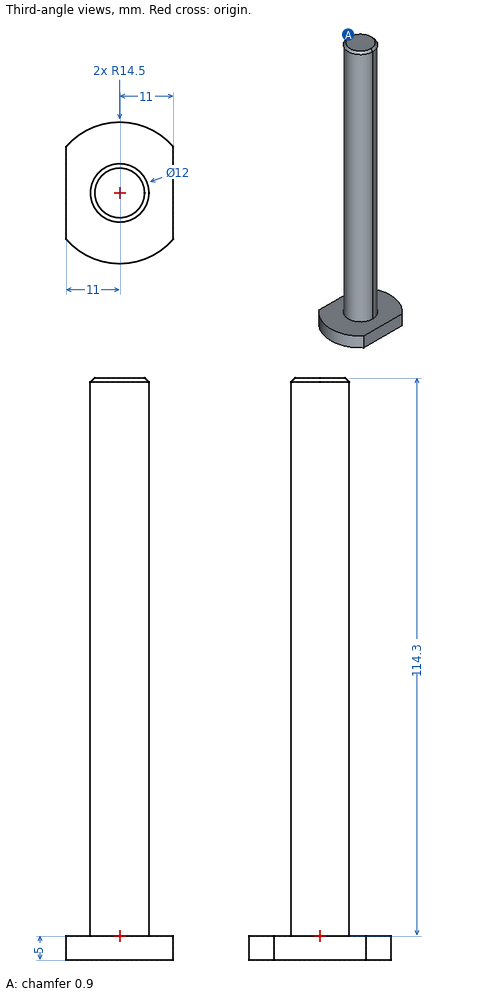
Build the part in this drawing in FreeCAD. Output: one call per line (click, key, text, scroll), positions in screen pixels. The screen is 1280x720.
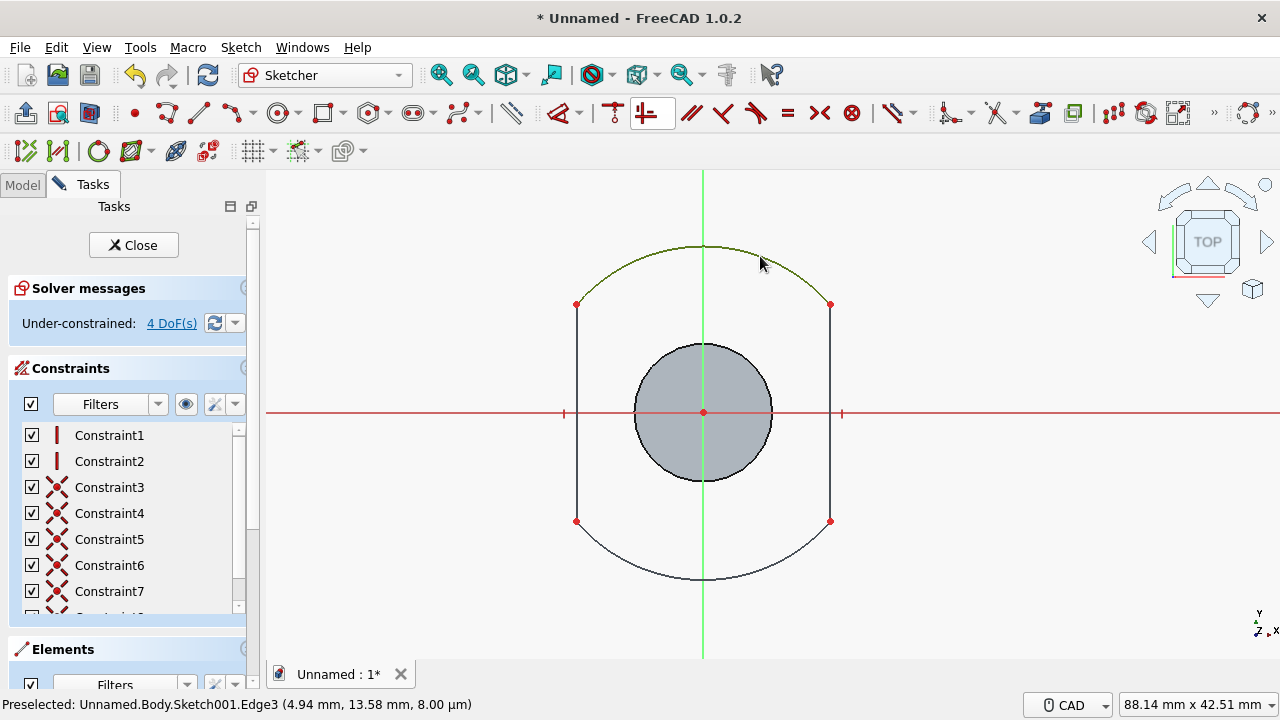
click(647, 570)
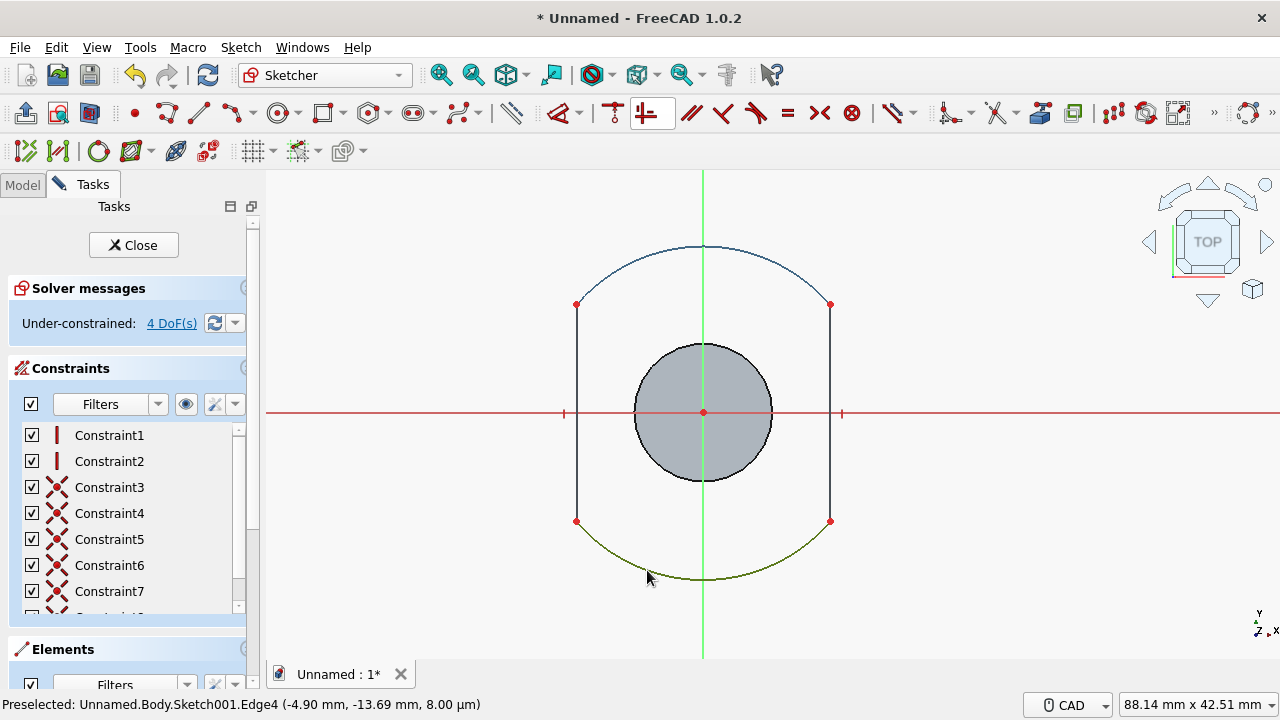
click(788, 114)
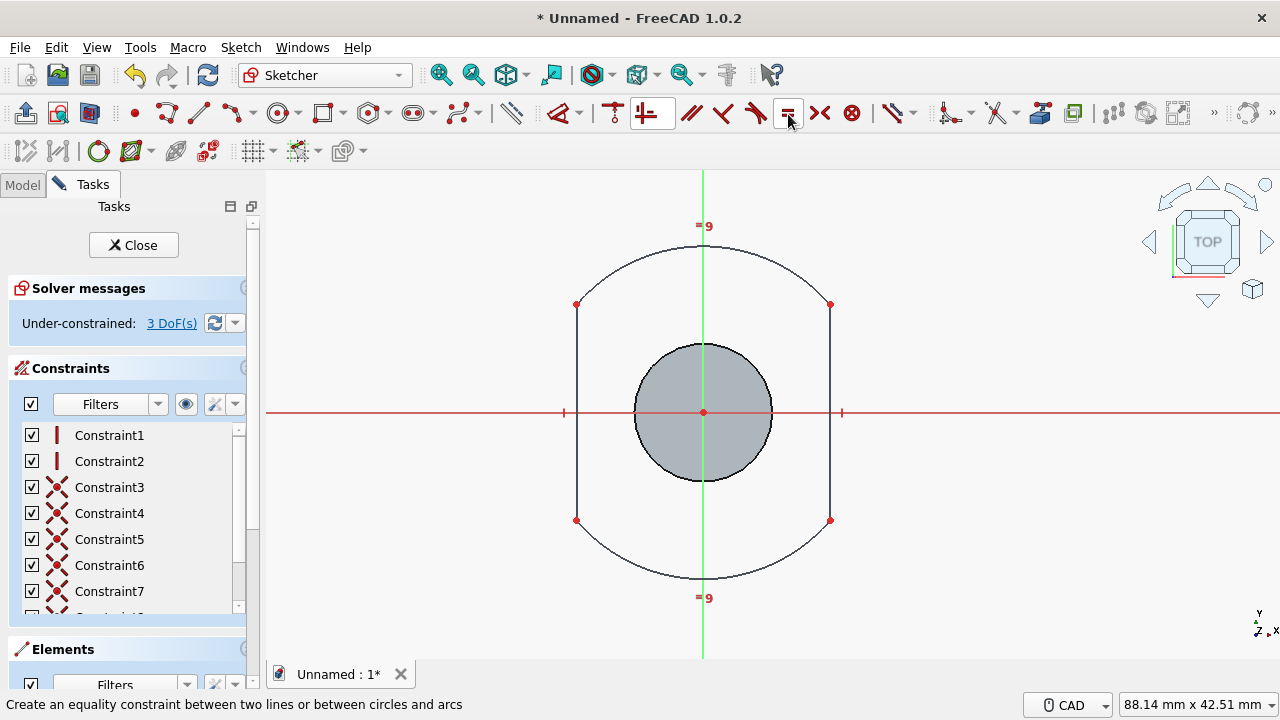
click(760, 256)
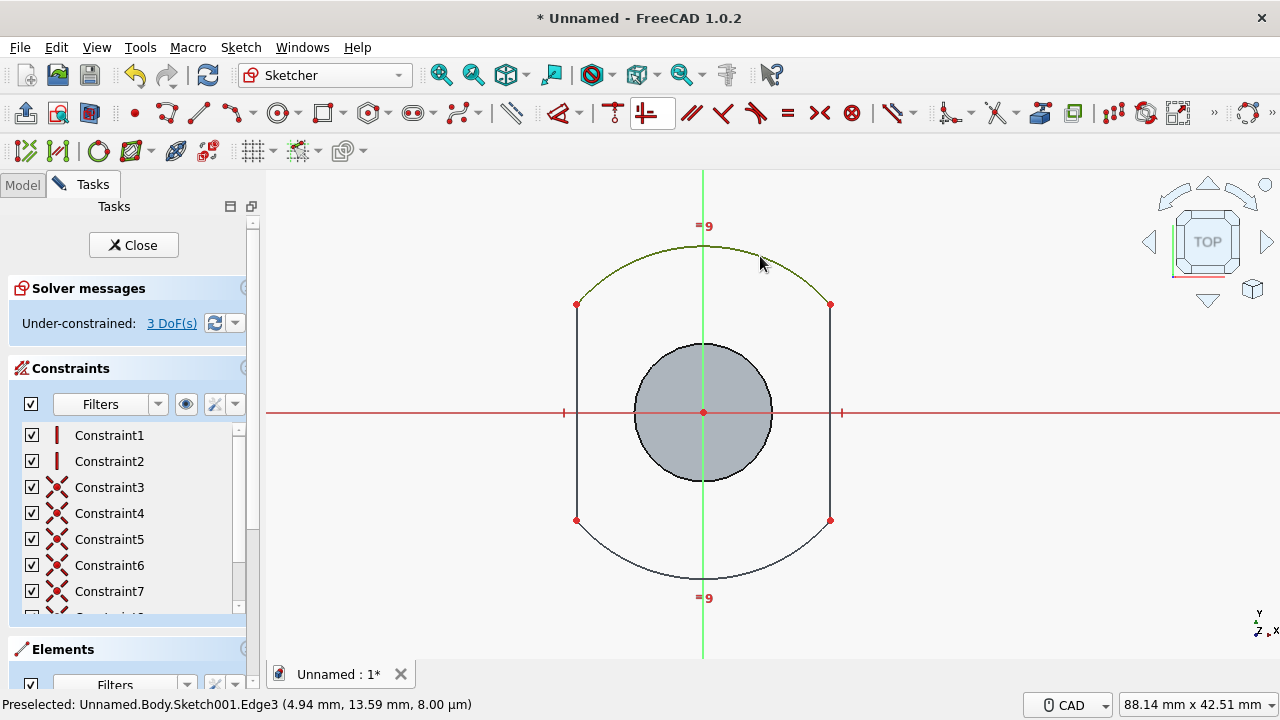
click(582, 114)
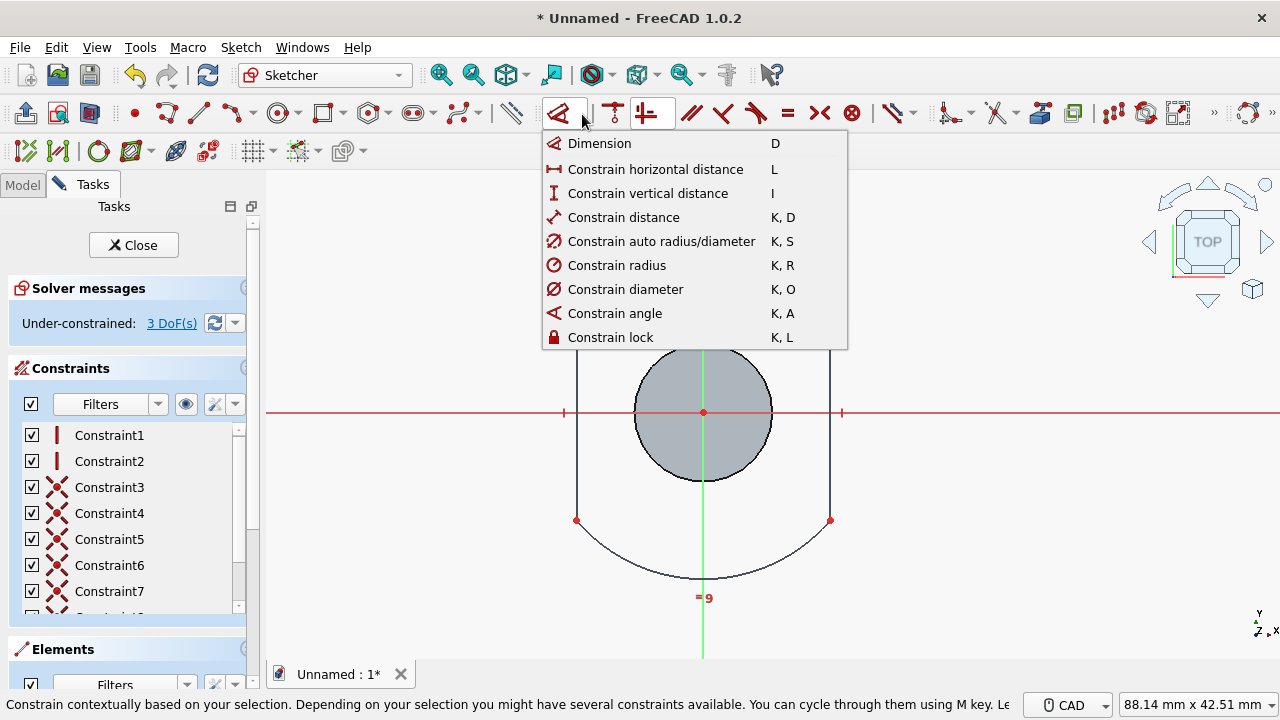
click(695, 265)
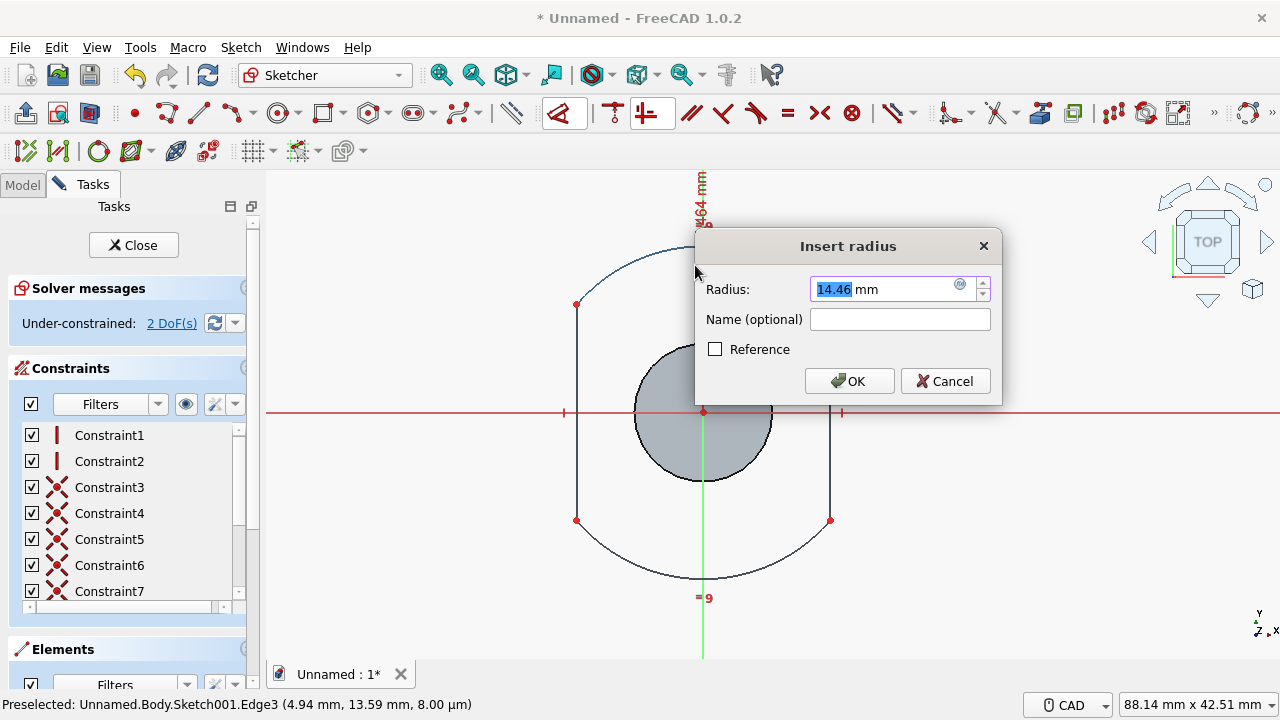
text(14.5)
key(Return)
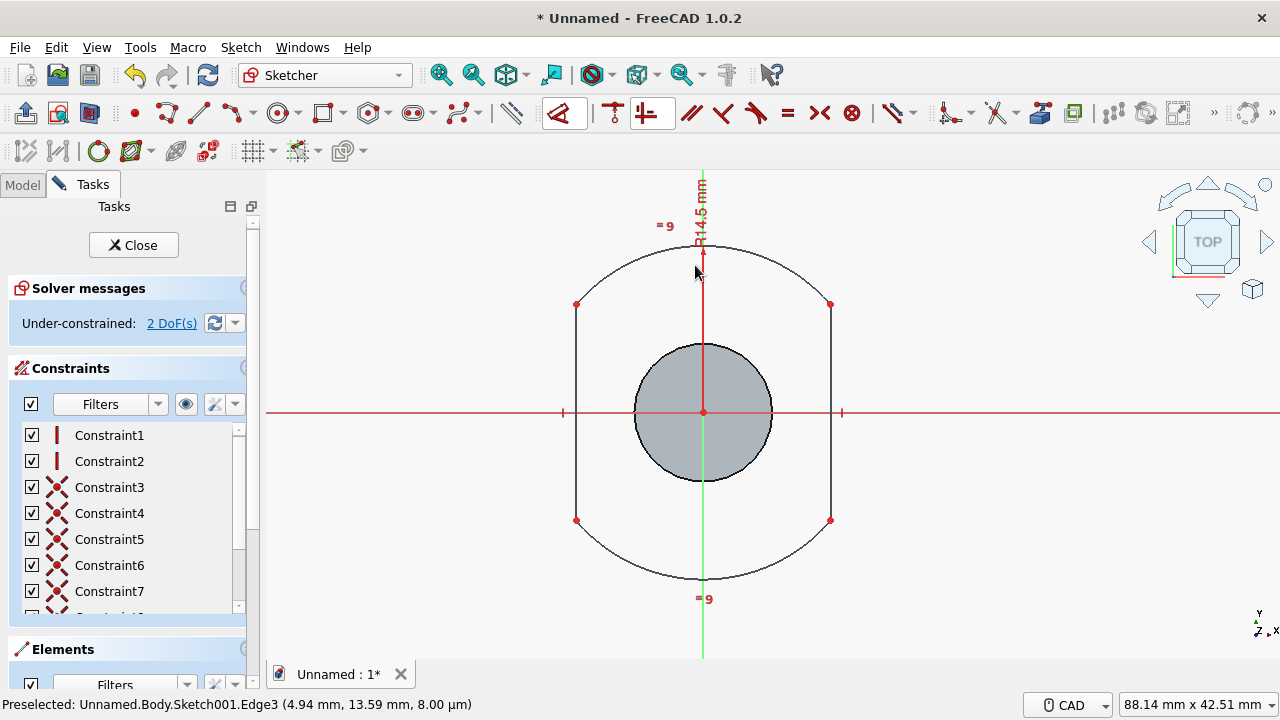
click(576, 521)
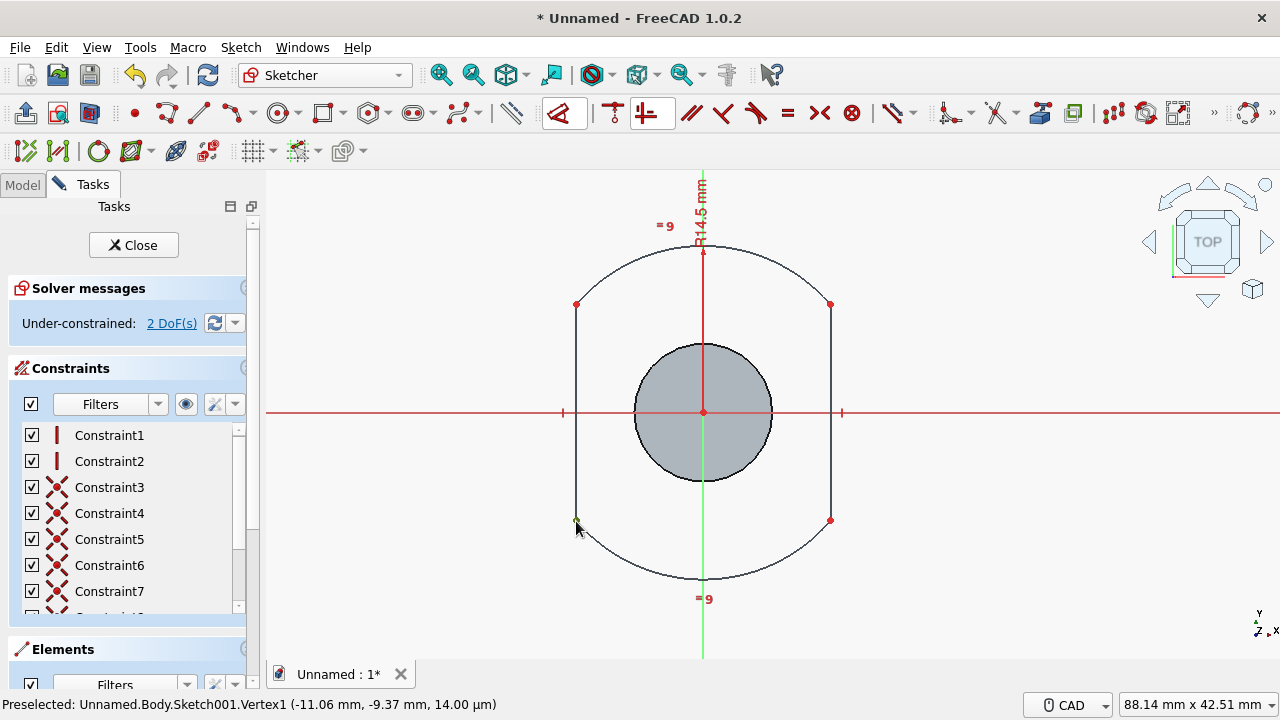
click(582, 114)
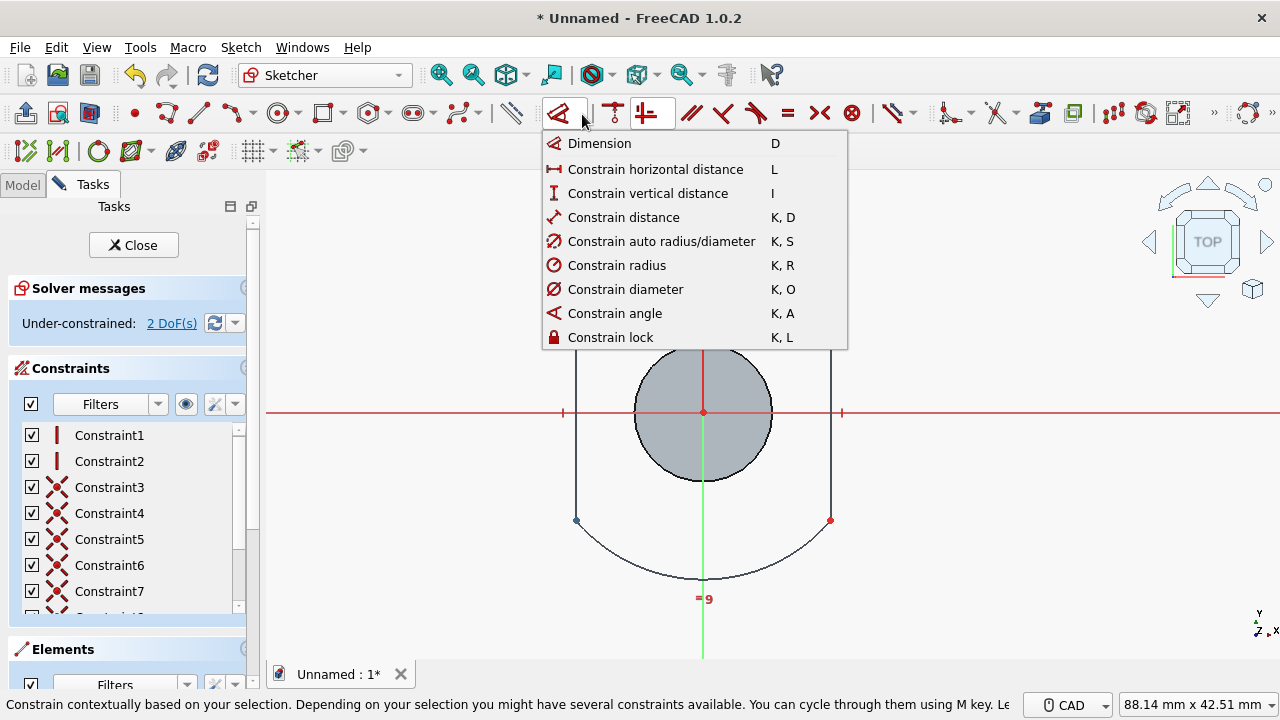
click(695, 169)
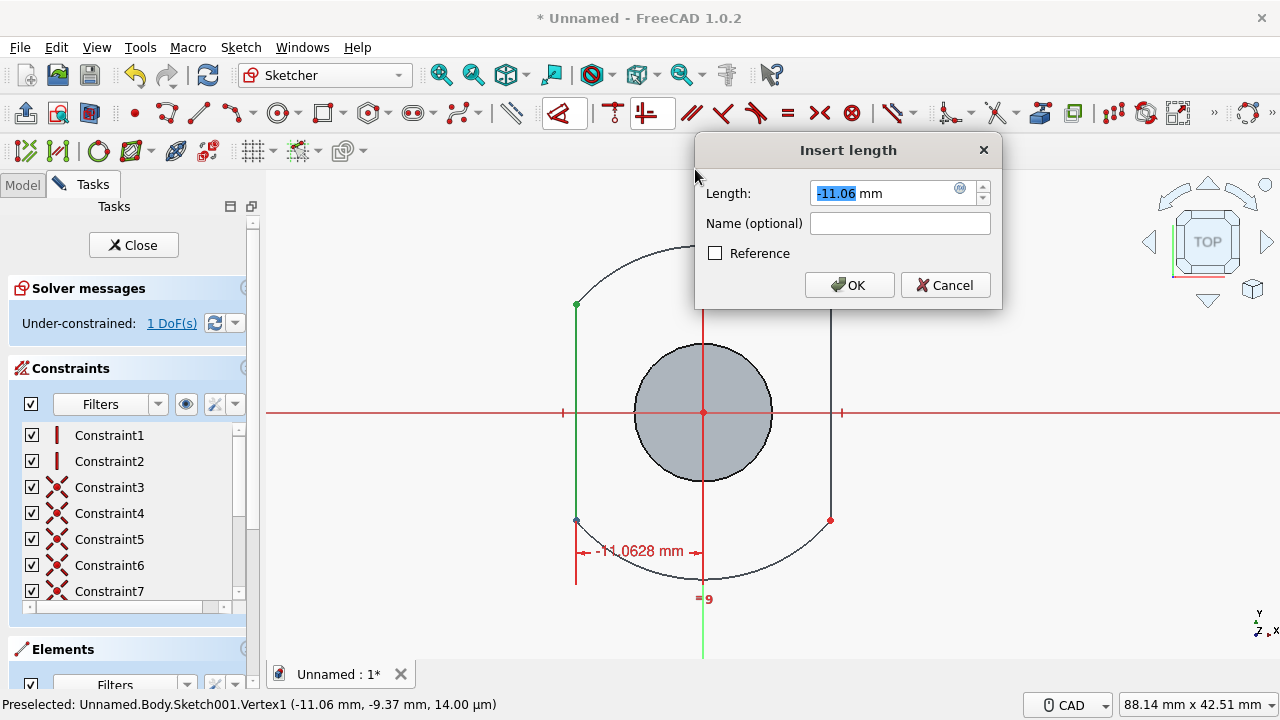
text(-11)
key(Return)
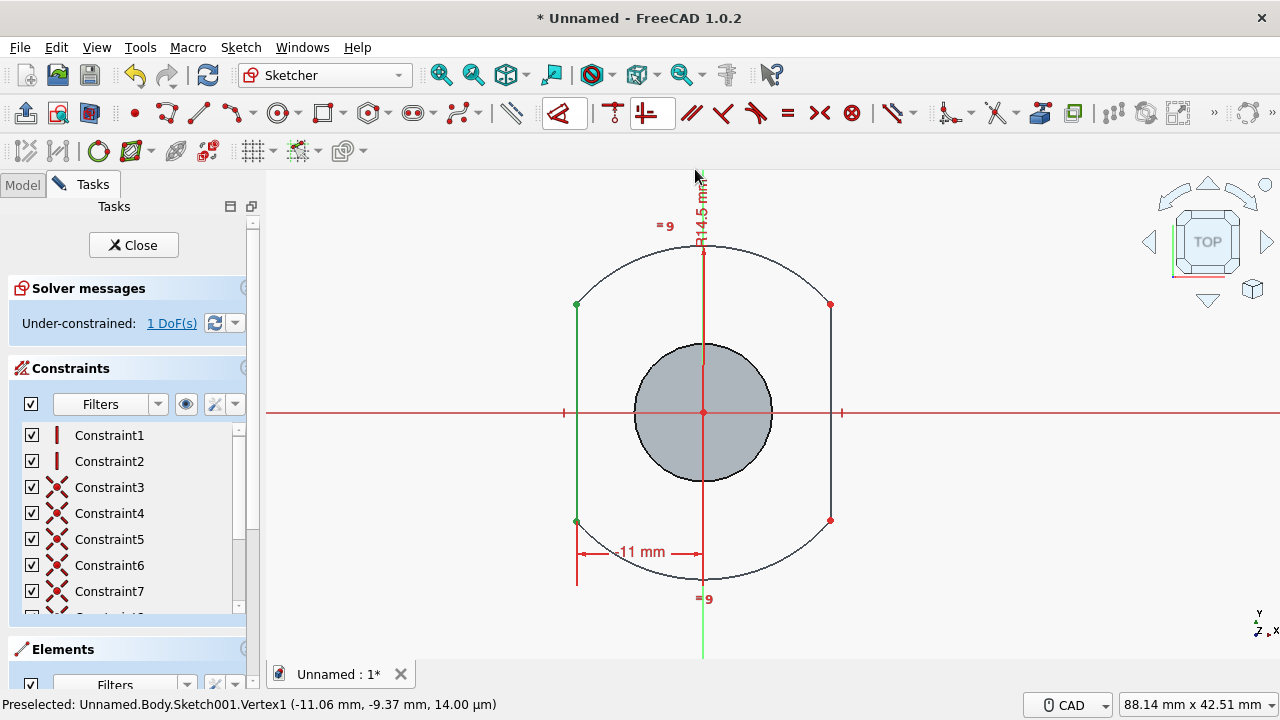
click(831, 305)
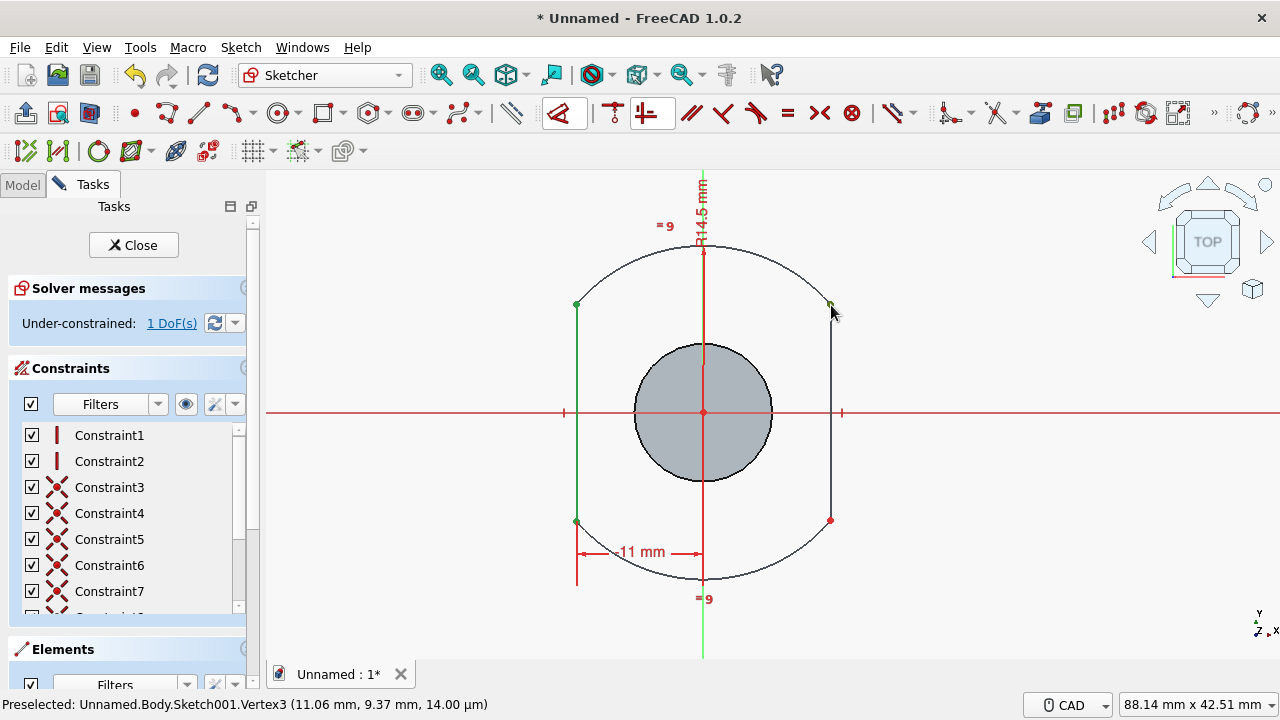
click(582, 114)